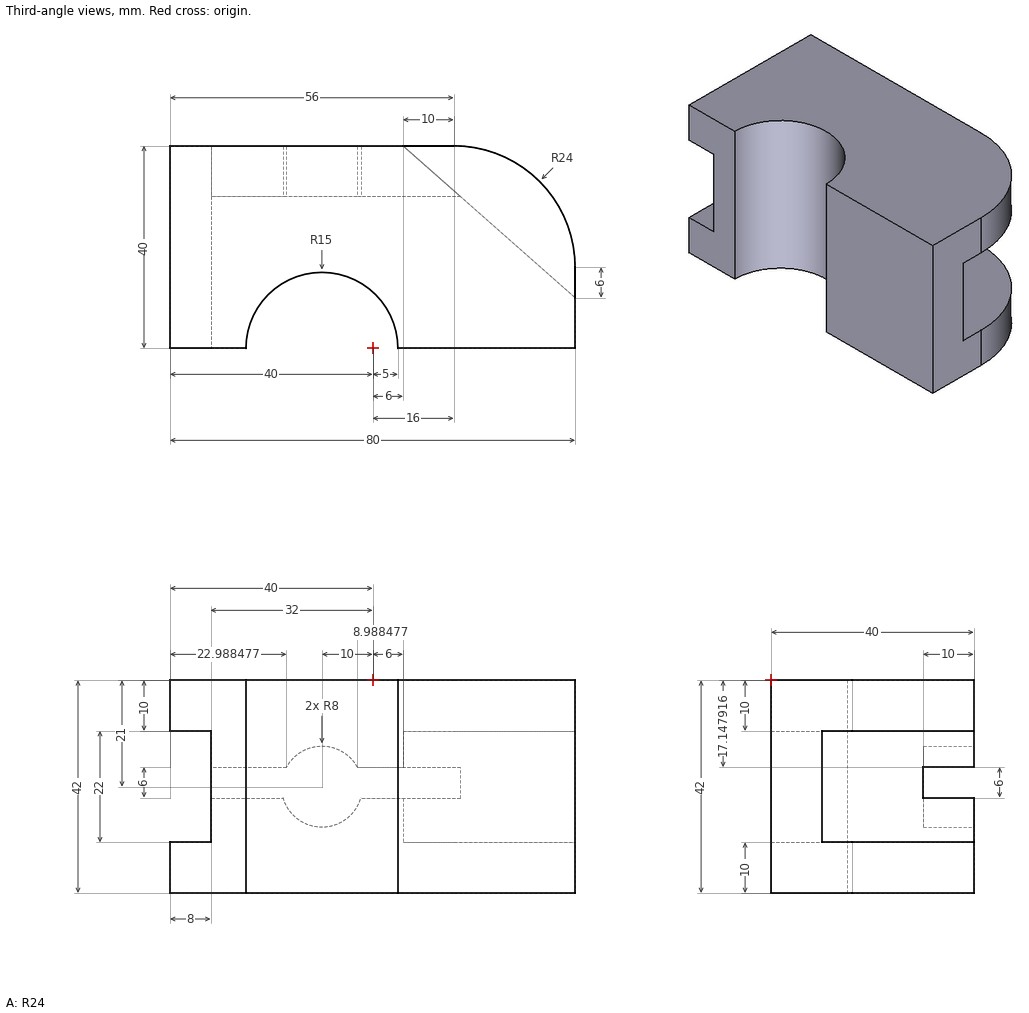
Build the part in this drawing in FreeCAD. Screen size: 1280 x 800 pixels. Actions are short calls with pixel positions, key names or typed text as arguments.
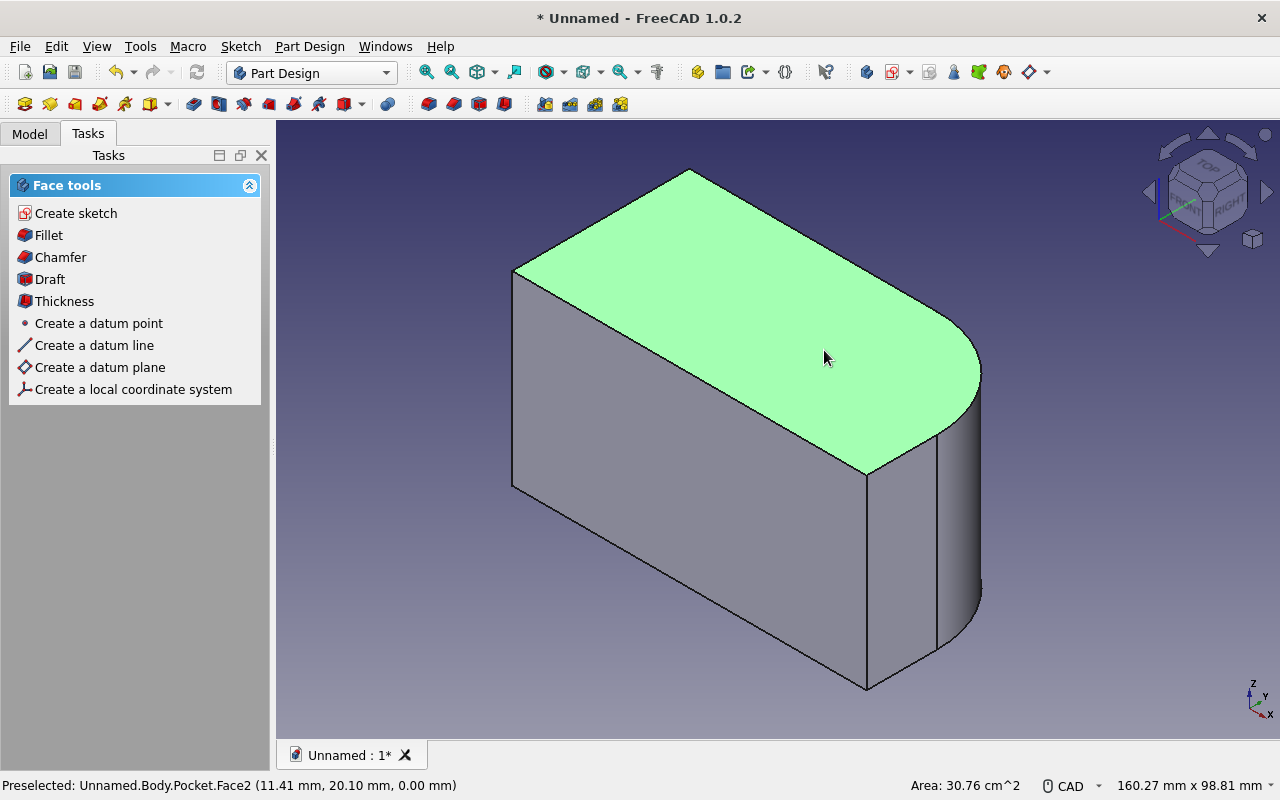
click(892, 72)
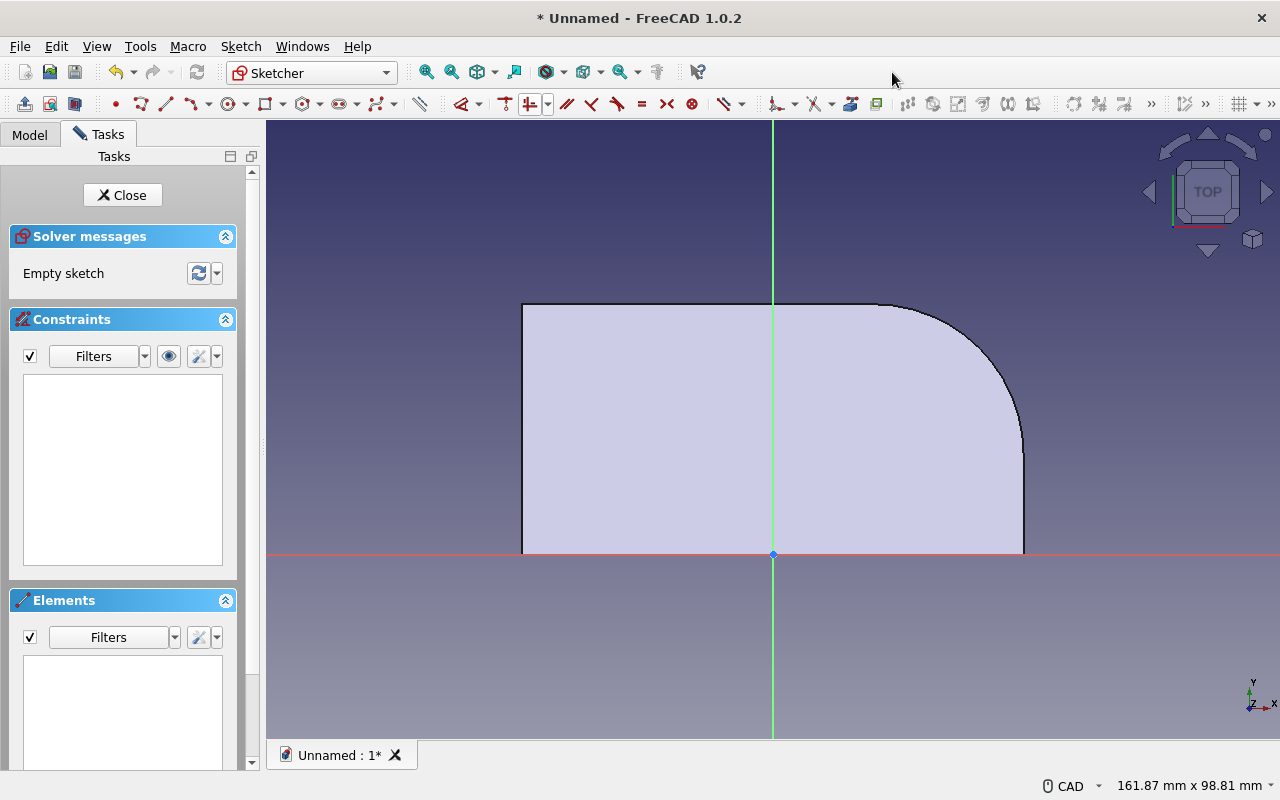
scroll(1115, 429, up, 2)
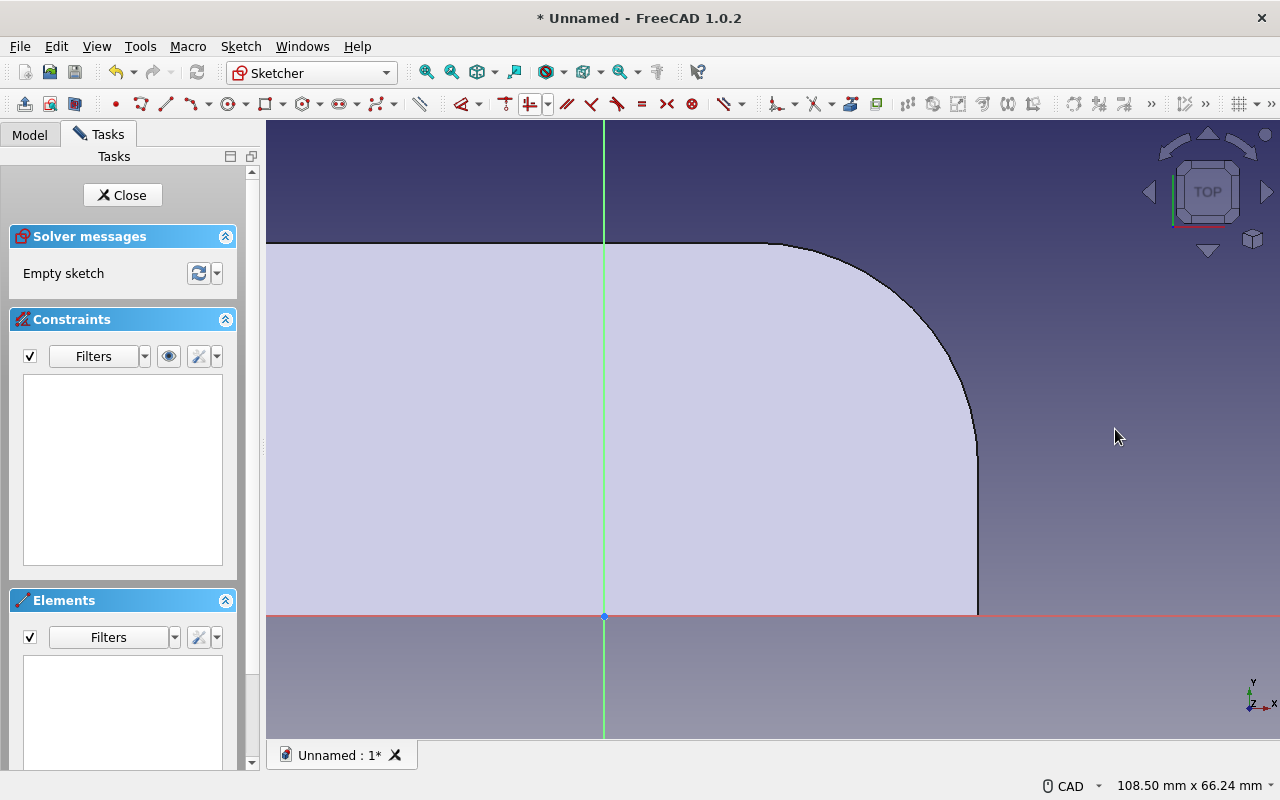
click(141, 104)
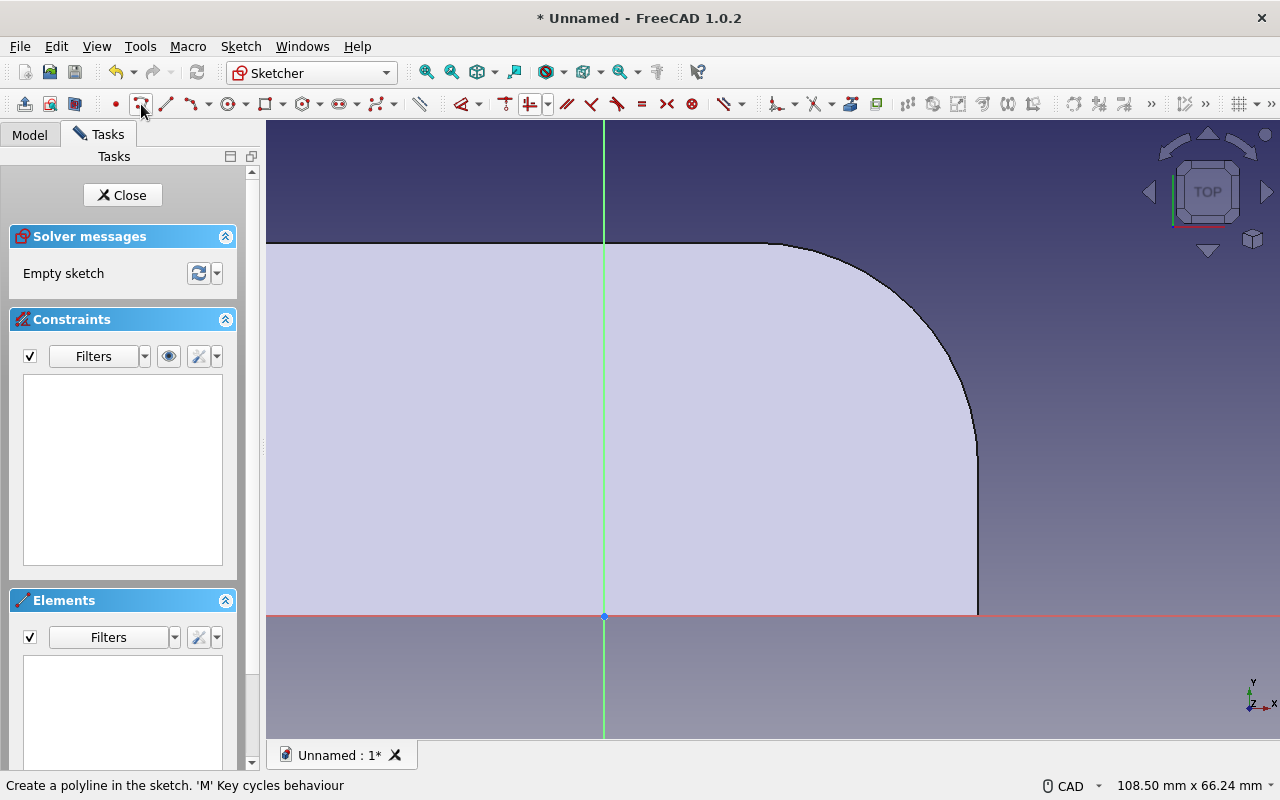
click(754, 243)
click(660, 243)
click(978, 523)
click(978, 467)
right_click(978, 467)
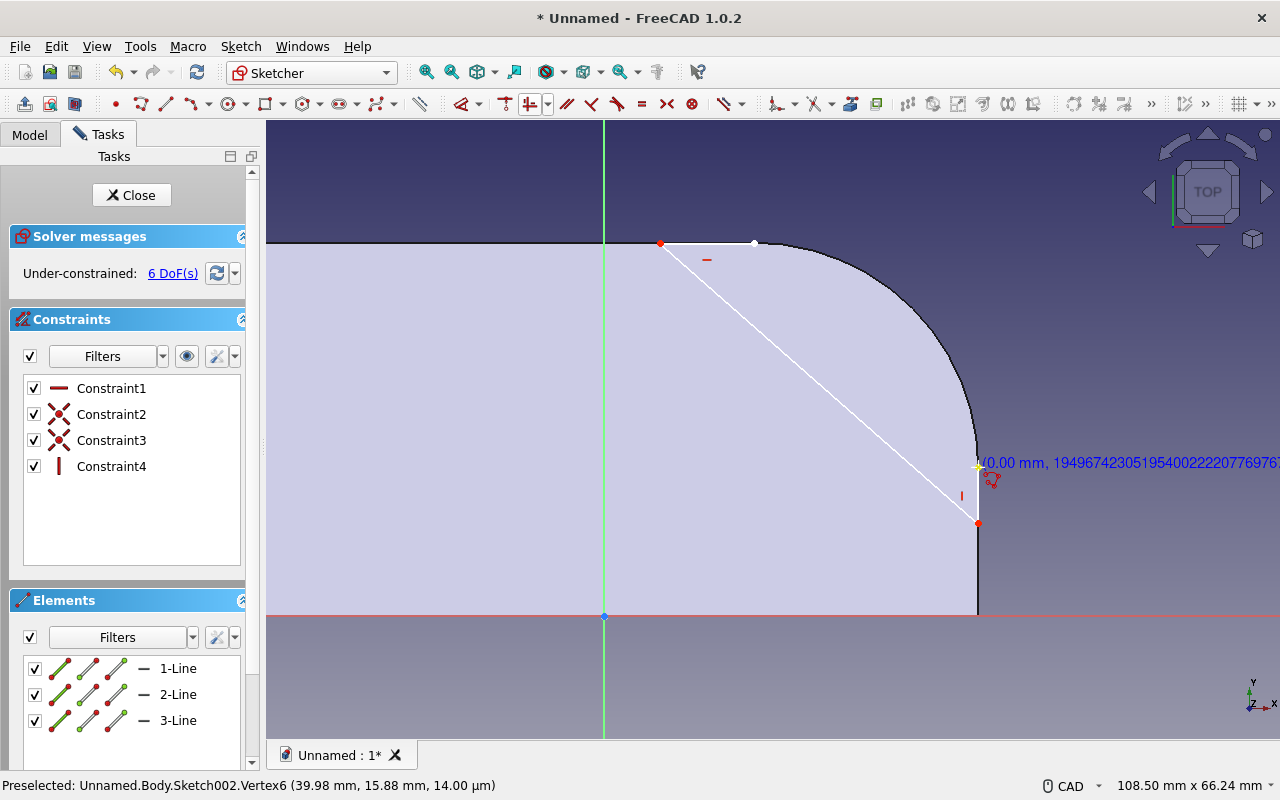
click(190, 104)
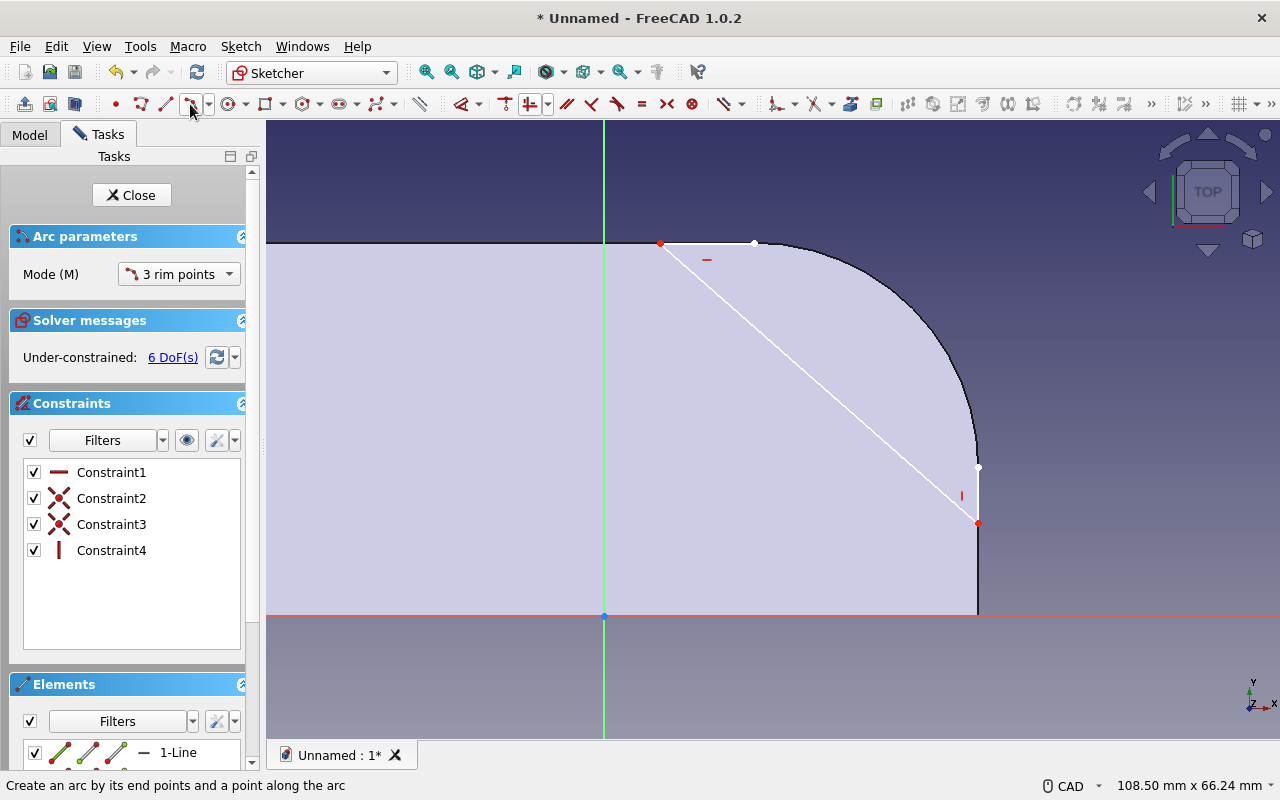
click(978, 468)
click(754, 244)
click(913, 308)
key(Escape)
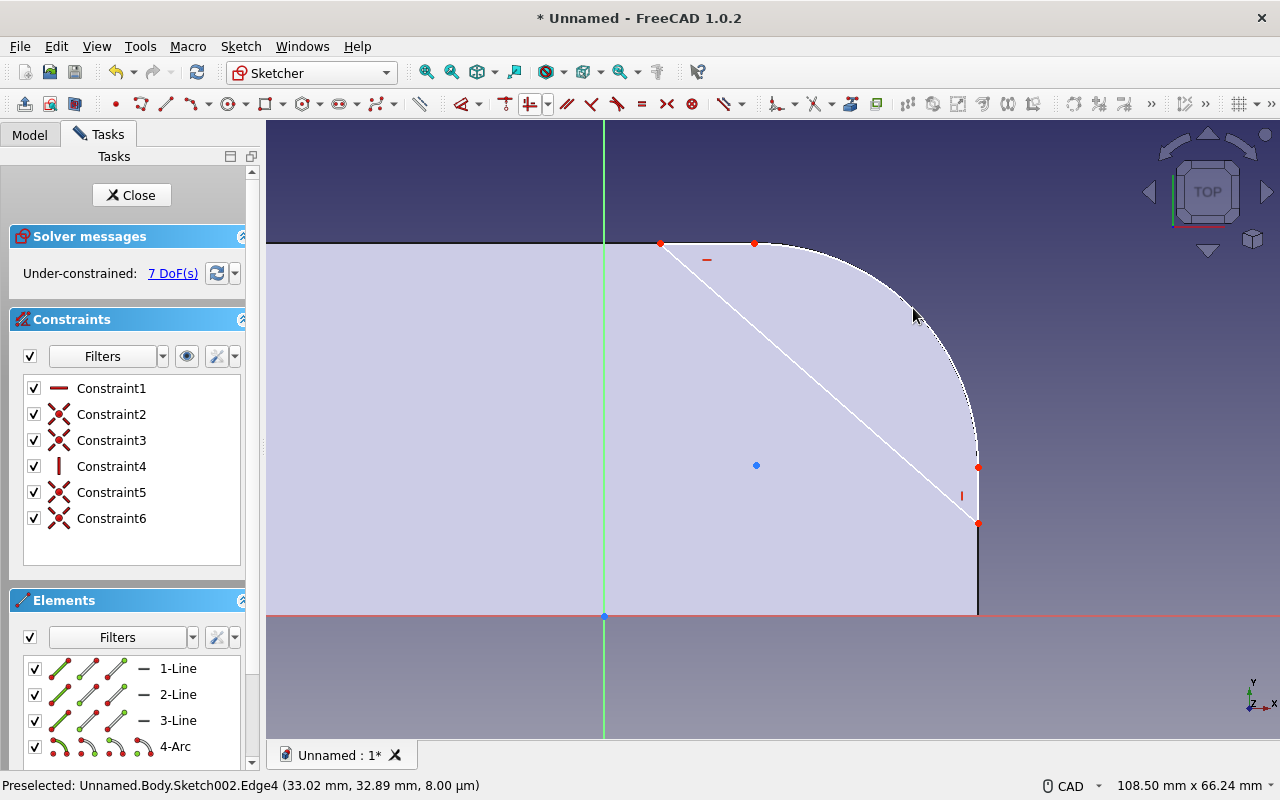
click(726, 244)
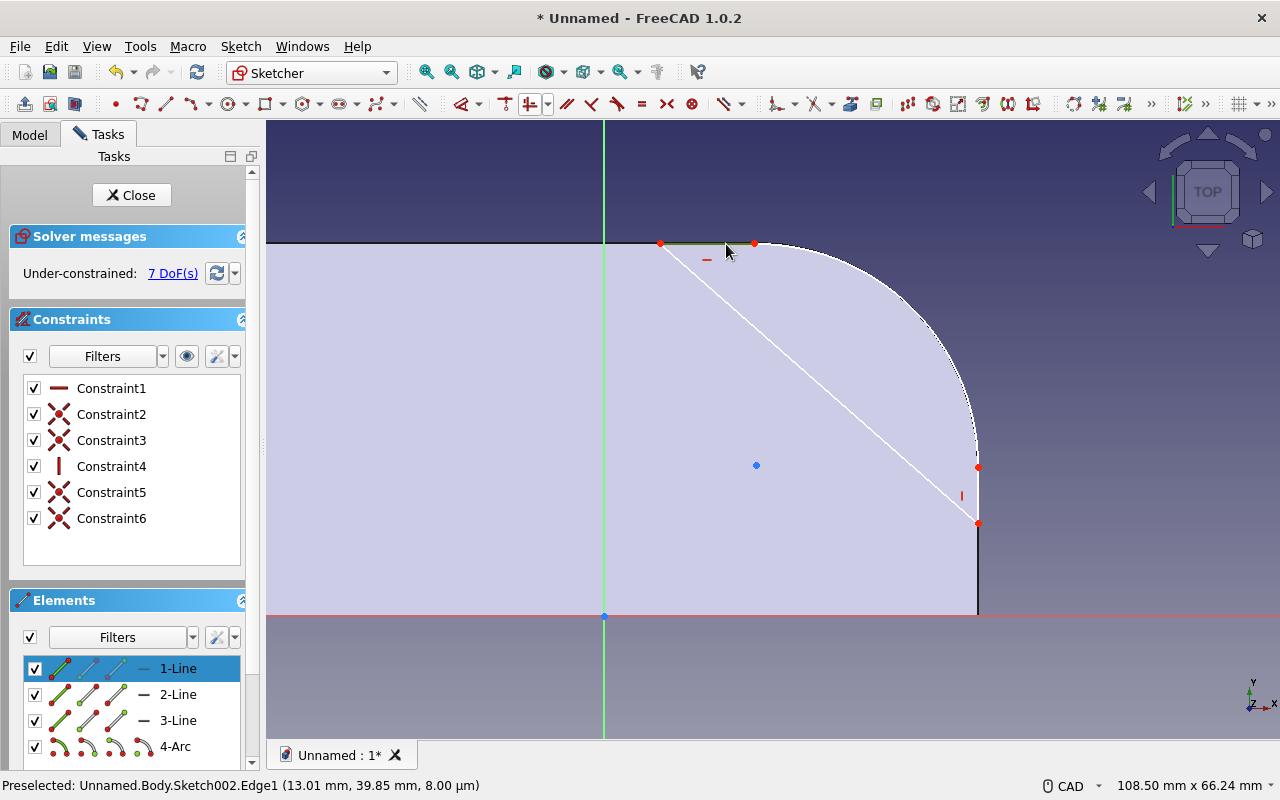
click(954, 366)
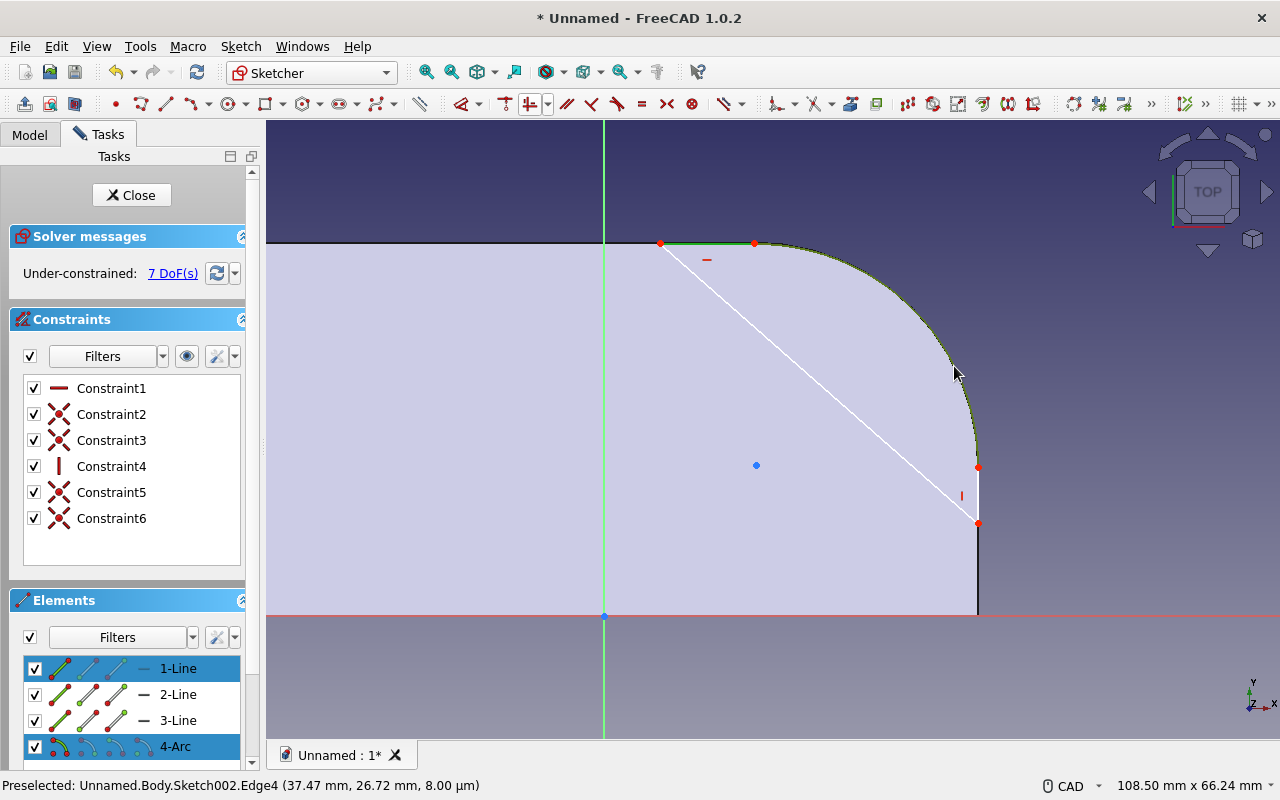
key(t)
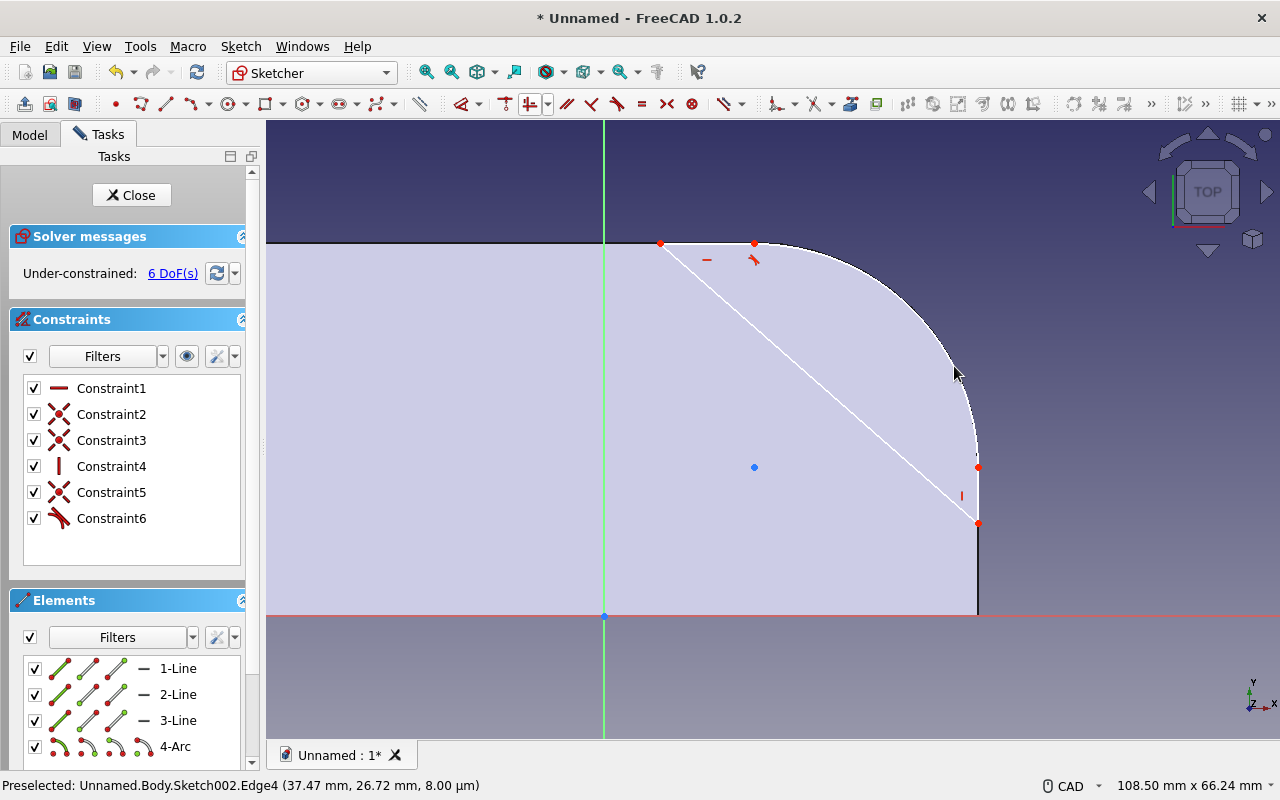
click(978, 507)